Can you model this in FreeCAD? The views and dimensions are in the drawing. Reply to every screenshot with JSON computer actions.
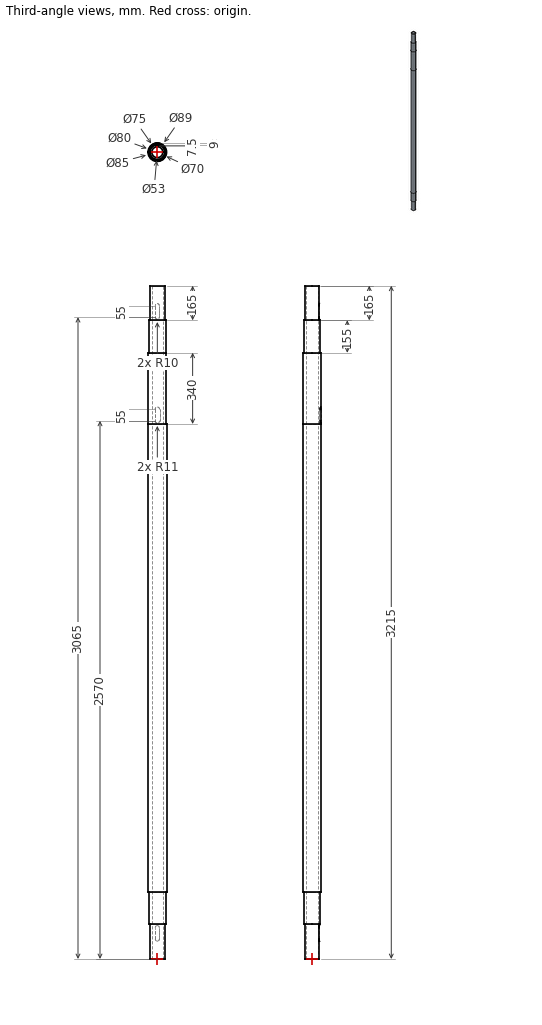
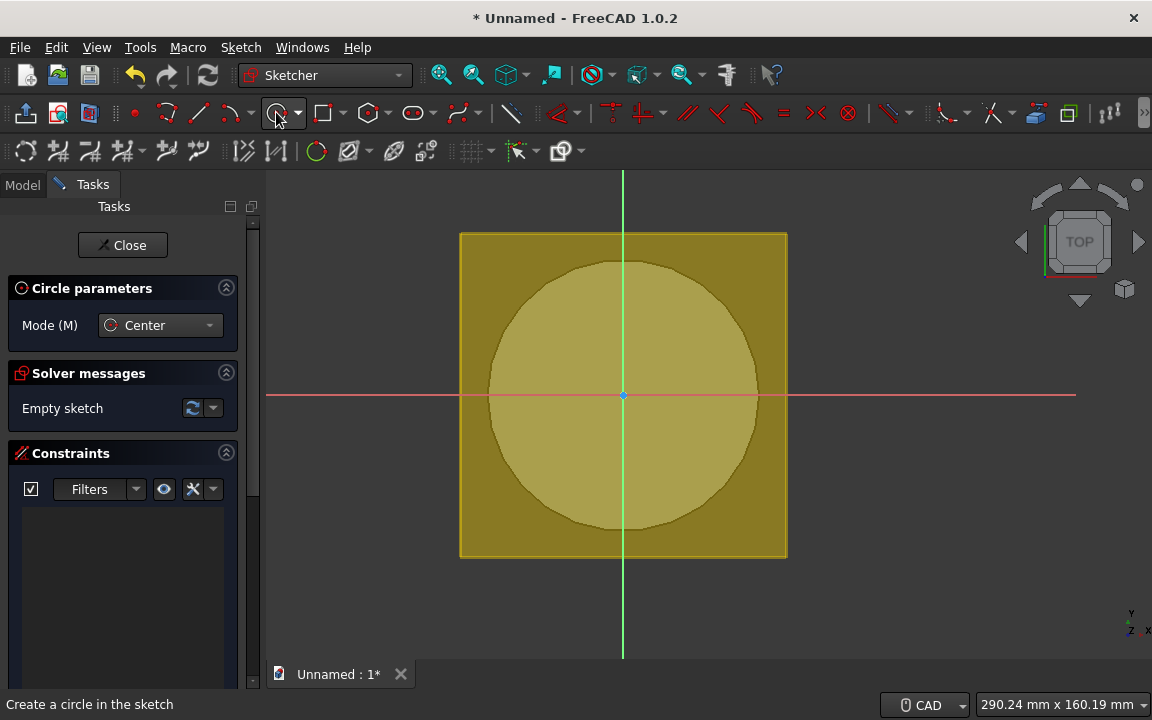
{"action": "left_click", "coordinate": [623, 395]}
{"action": "mouse_move", "coordinate": [719, 299]}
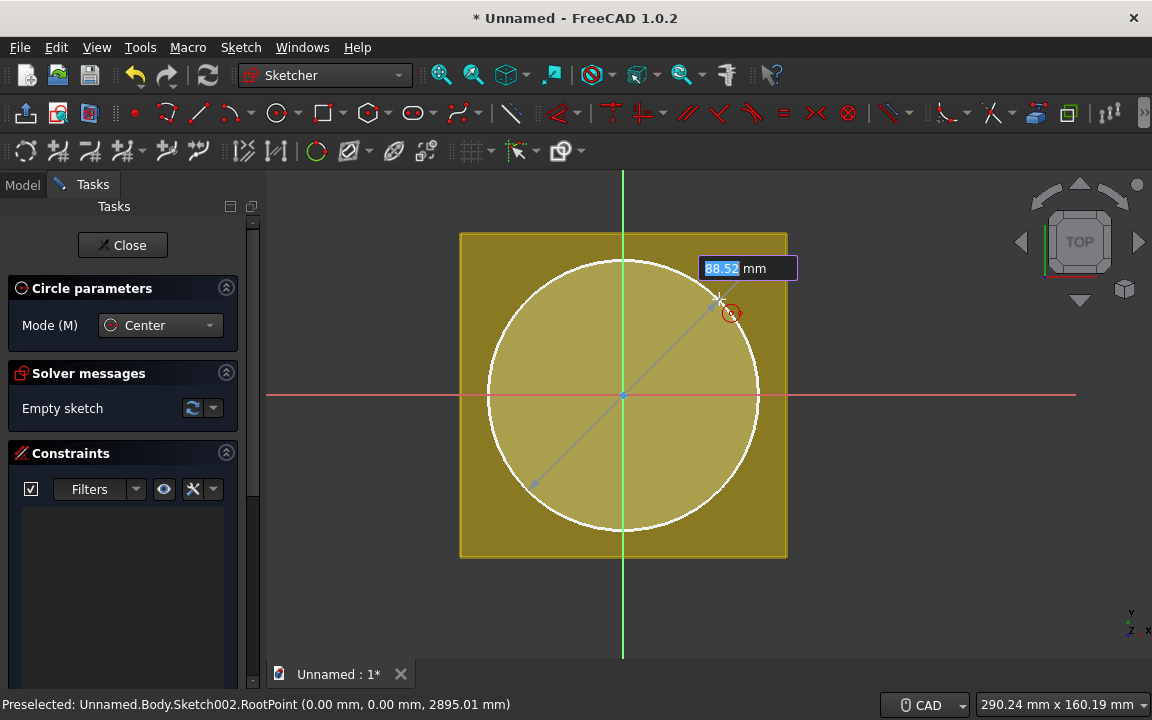
{"action": "type", "text": "89"}
{"action": "key", "text": "Return"}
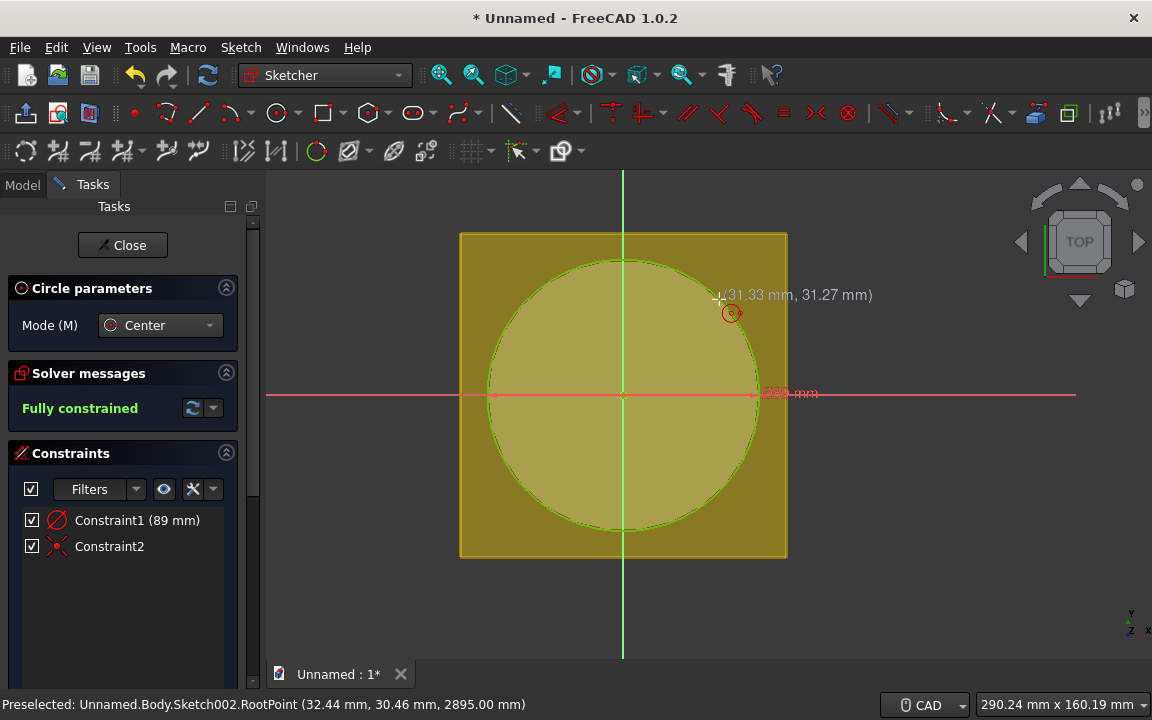
{"action": "left_click", "coordinate": [623, 395]}
{"action": "mouse_move", "coordinate": [710, 309]}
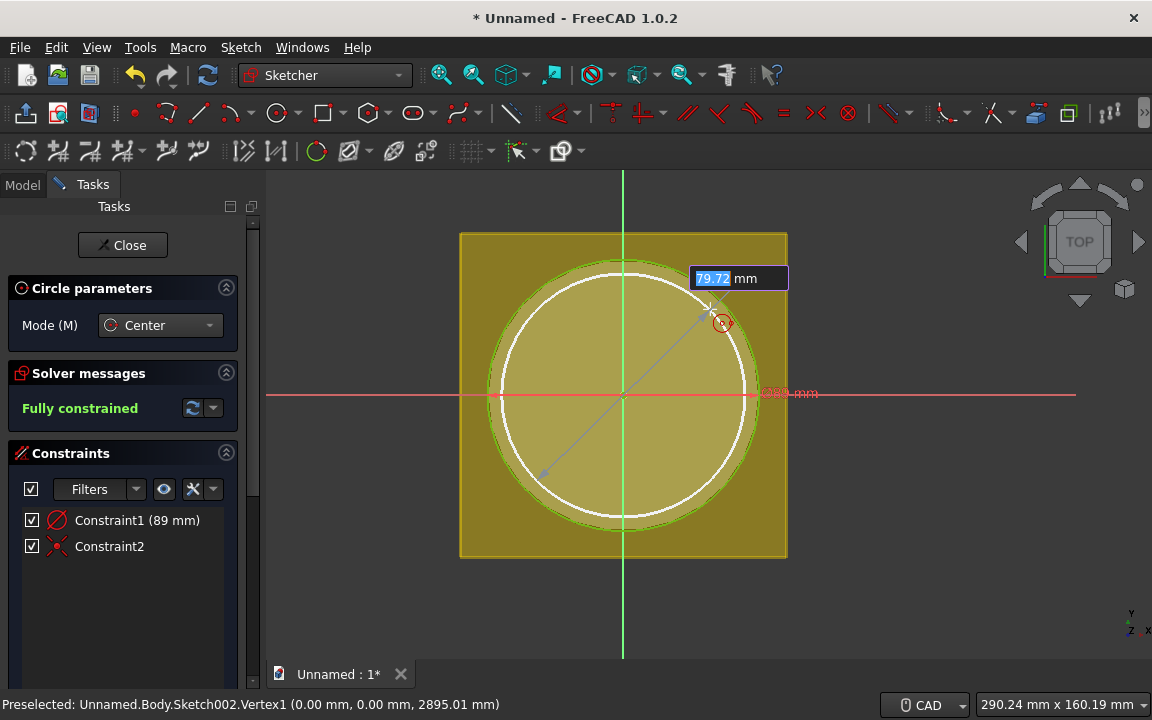
{"action": "type", "text": "80"}
{"action": "key", "text": "Return"}
{"action": "key", "text": "Escape"}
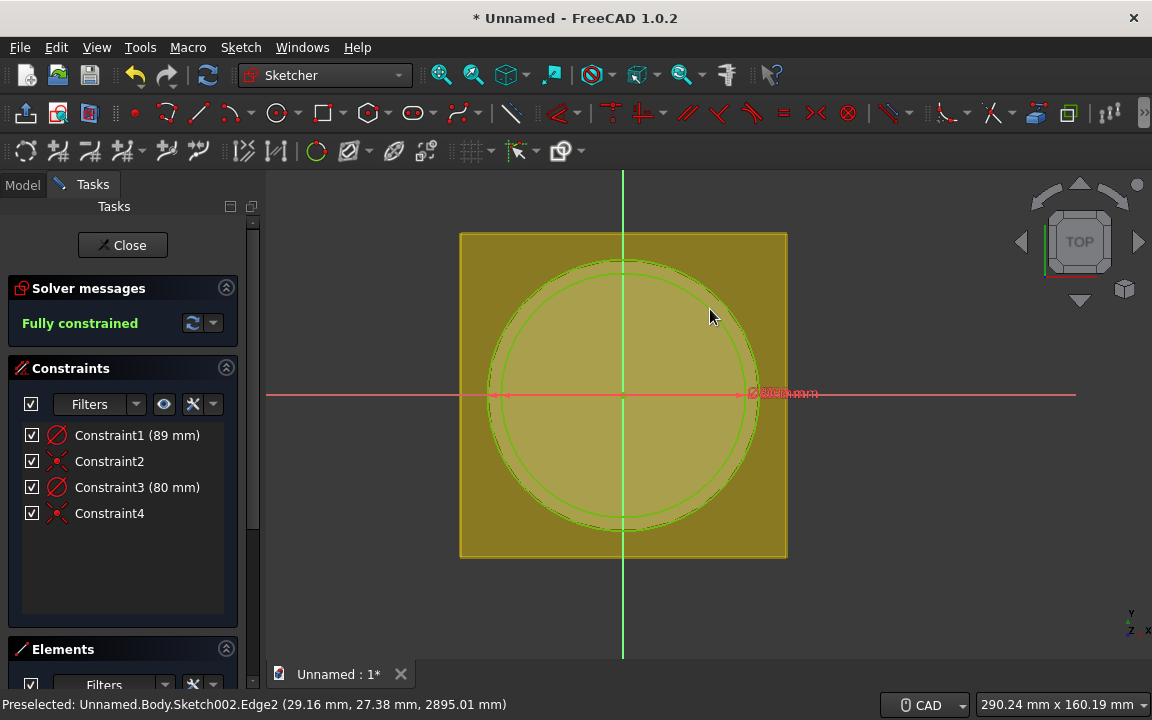
{"action": "left_click", "coordinate": [123, 245]}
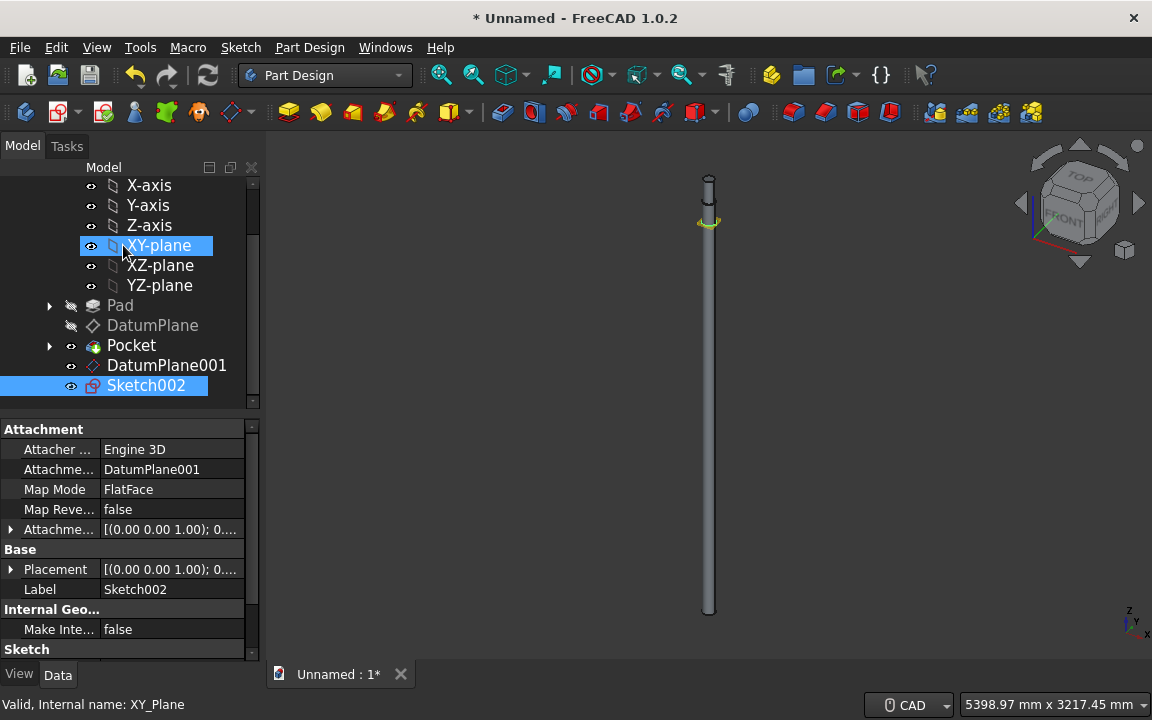
{"action": "left_click", "coordinate": [504, 112]}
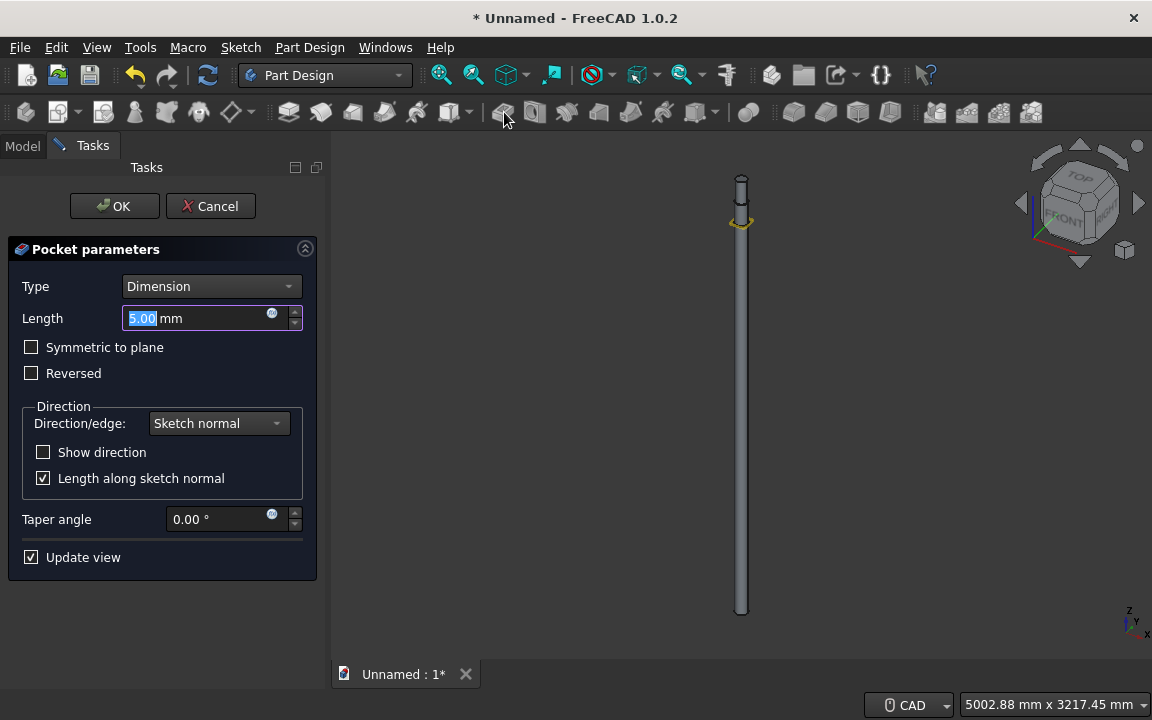
{"action": "type", "text": "155"}
{"action": "key", "text": "Tab"}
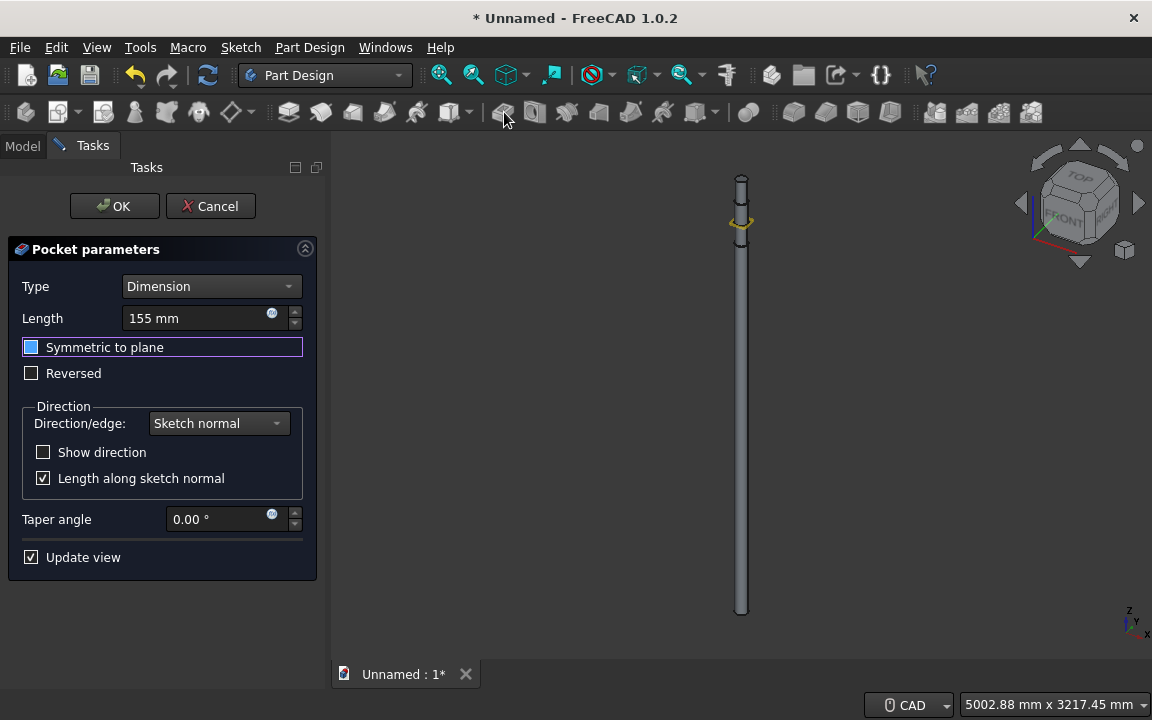
{"action": "left_click", "coordinate": [30, 373]}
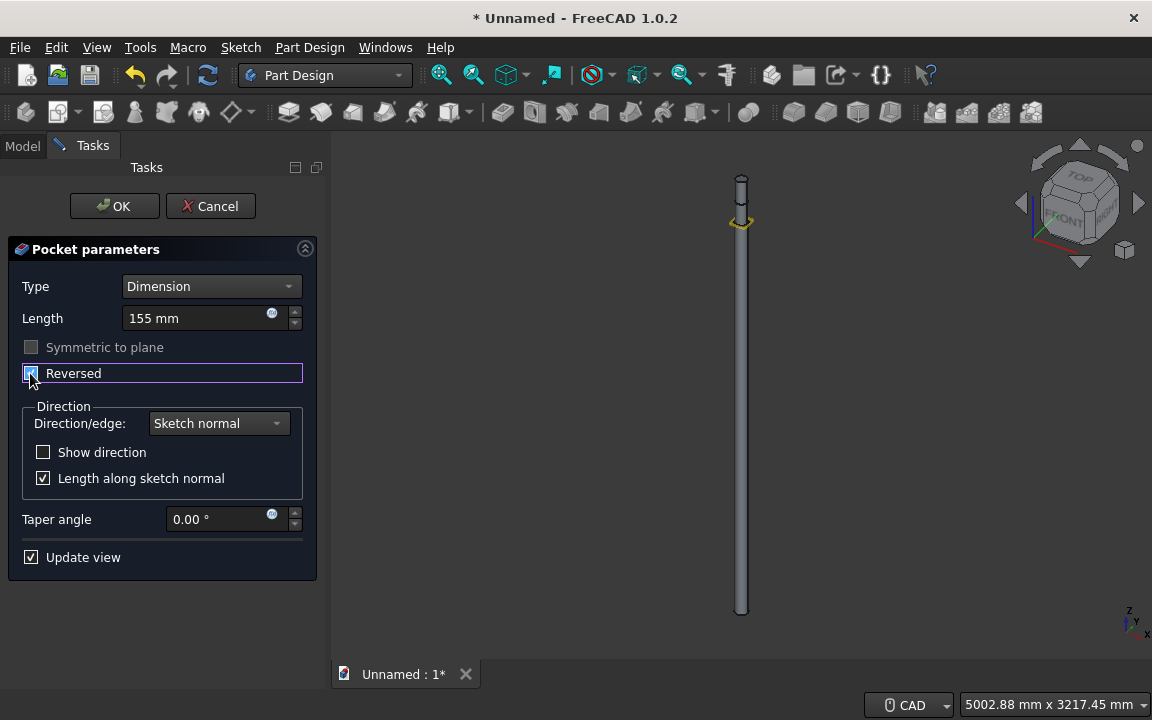
{"action": "left_click", "coordinate": [115, 206]}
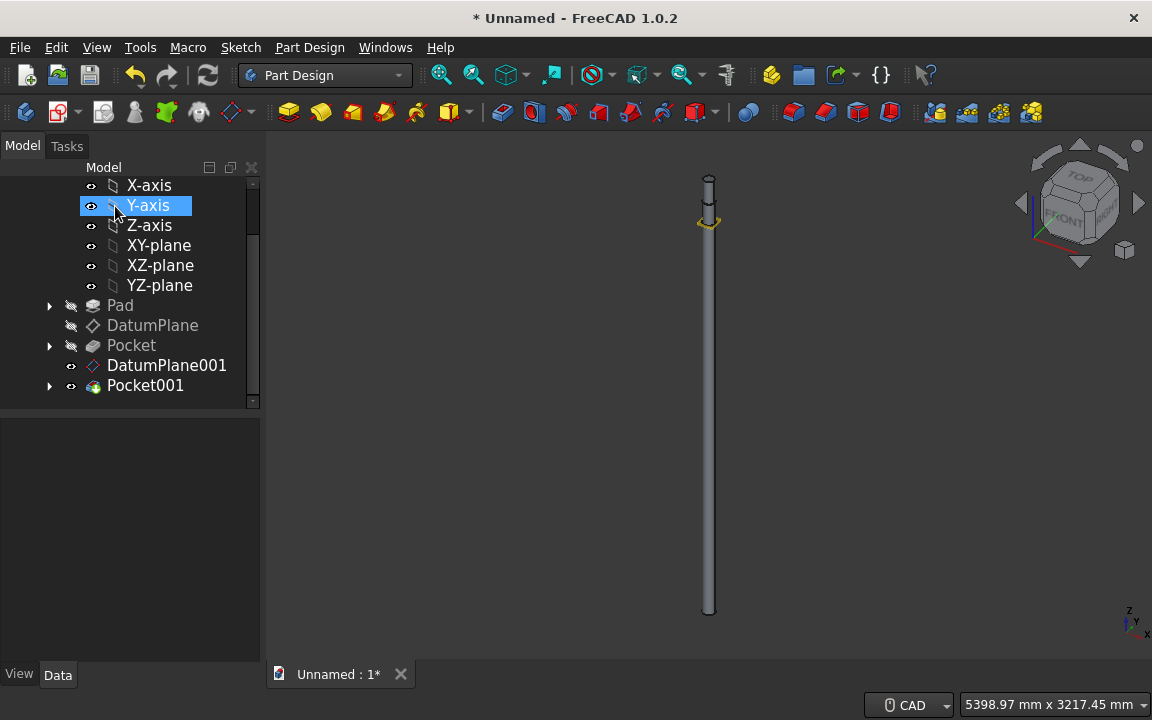
{"action": "left_click", "coordinate": [116, 366]}
{"action": "key", "text": "space"}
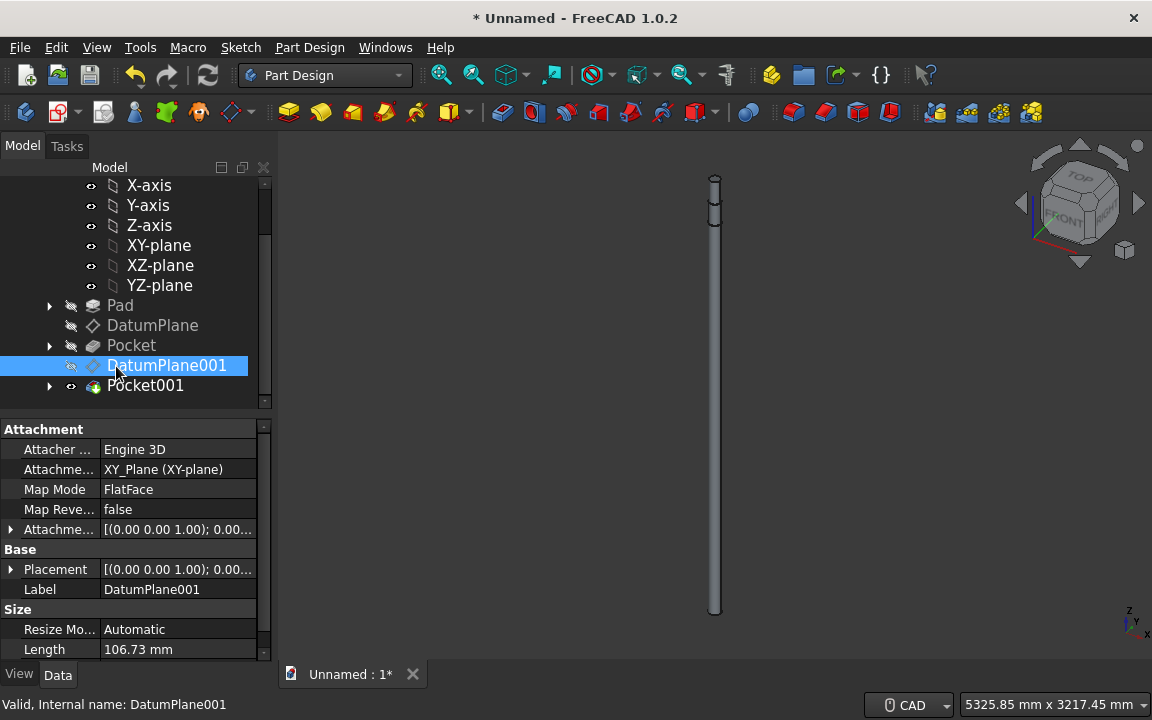
{"action": "scroll", "coordinate": [160, 281], "scroll_direction": "down", "scroll_amount": 3}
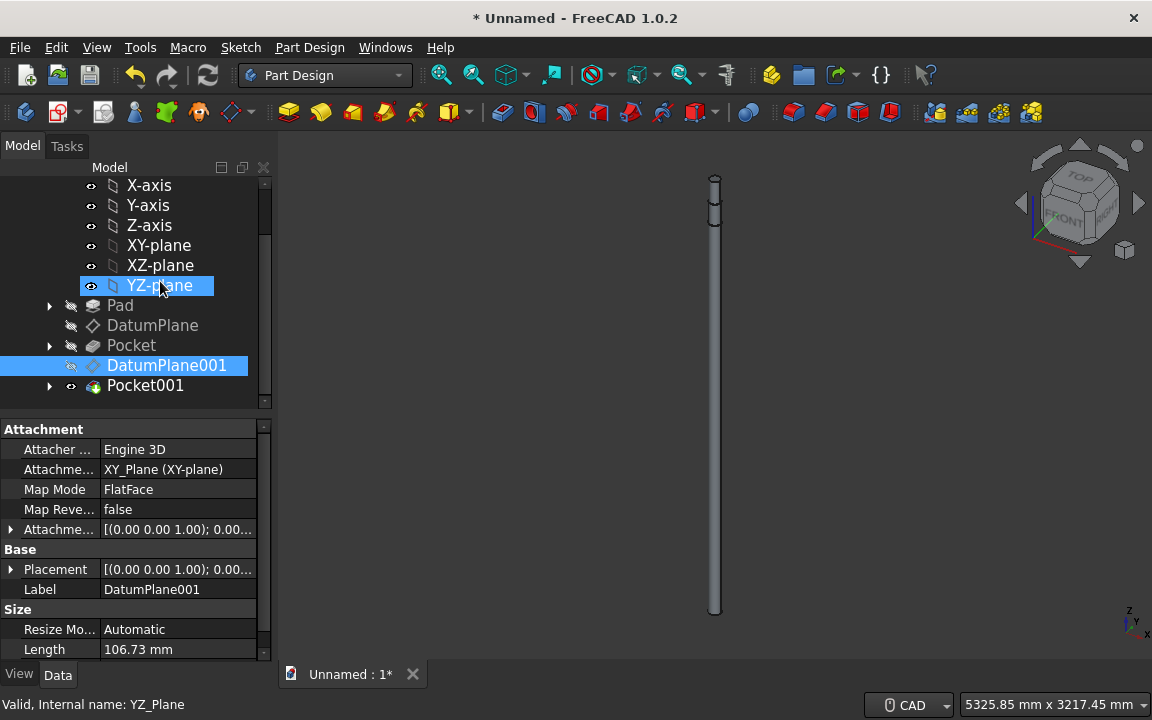
{"action": "scroll", "coordinate": [160, 281], "scroll_direction": "up", "scroll_amount": 15}